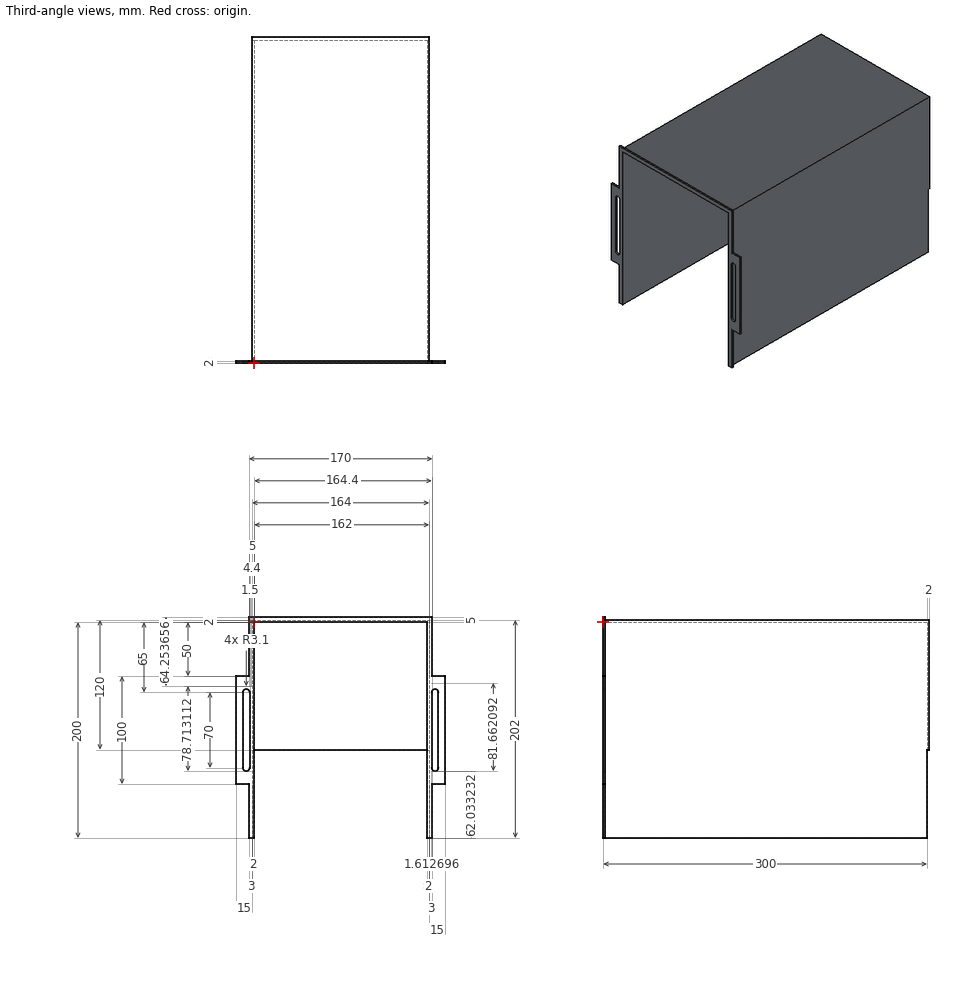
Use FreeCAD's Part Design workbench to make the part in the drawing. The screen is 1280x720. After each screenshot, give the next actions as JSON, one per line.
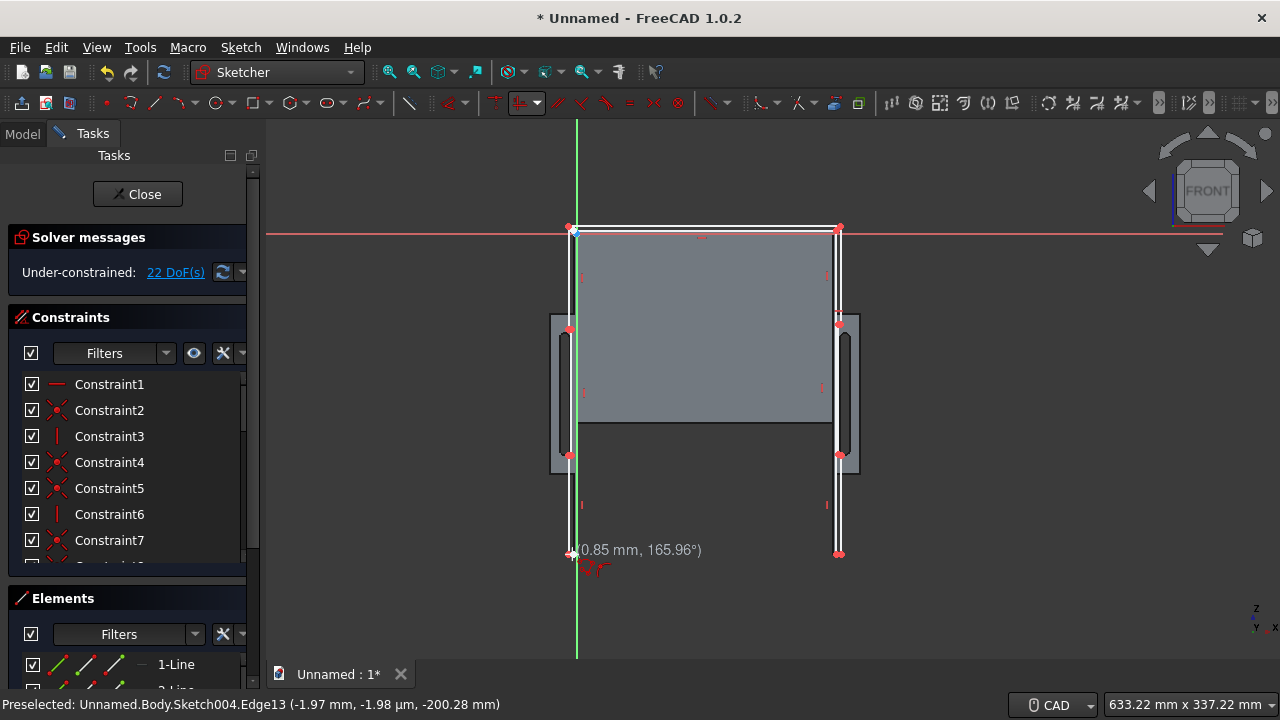
{"action": "scroll", "coordinate": [574, 231], "scroll_direction": "up", "scroll_amount": 9}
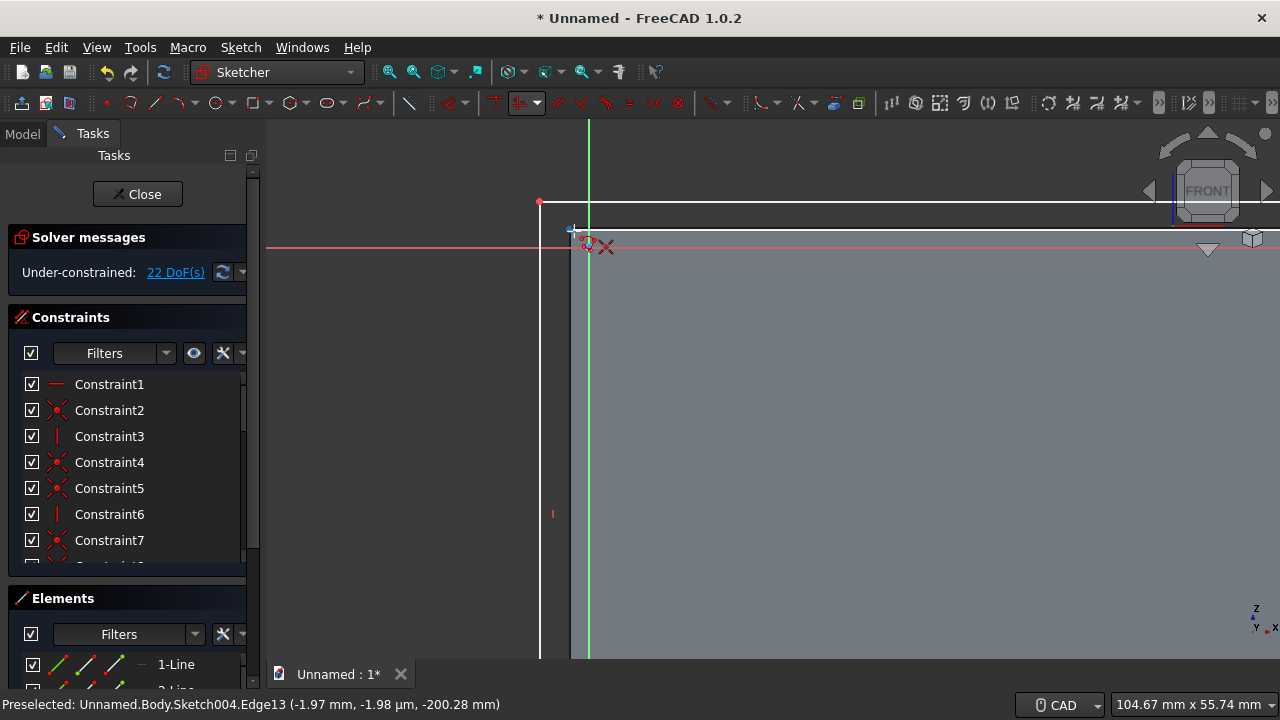
{"action": "left_click", "coordinate": [569, 230]}
{"action": "key", "text": "Escape"}
{"action": "key", "text": "Escape"}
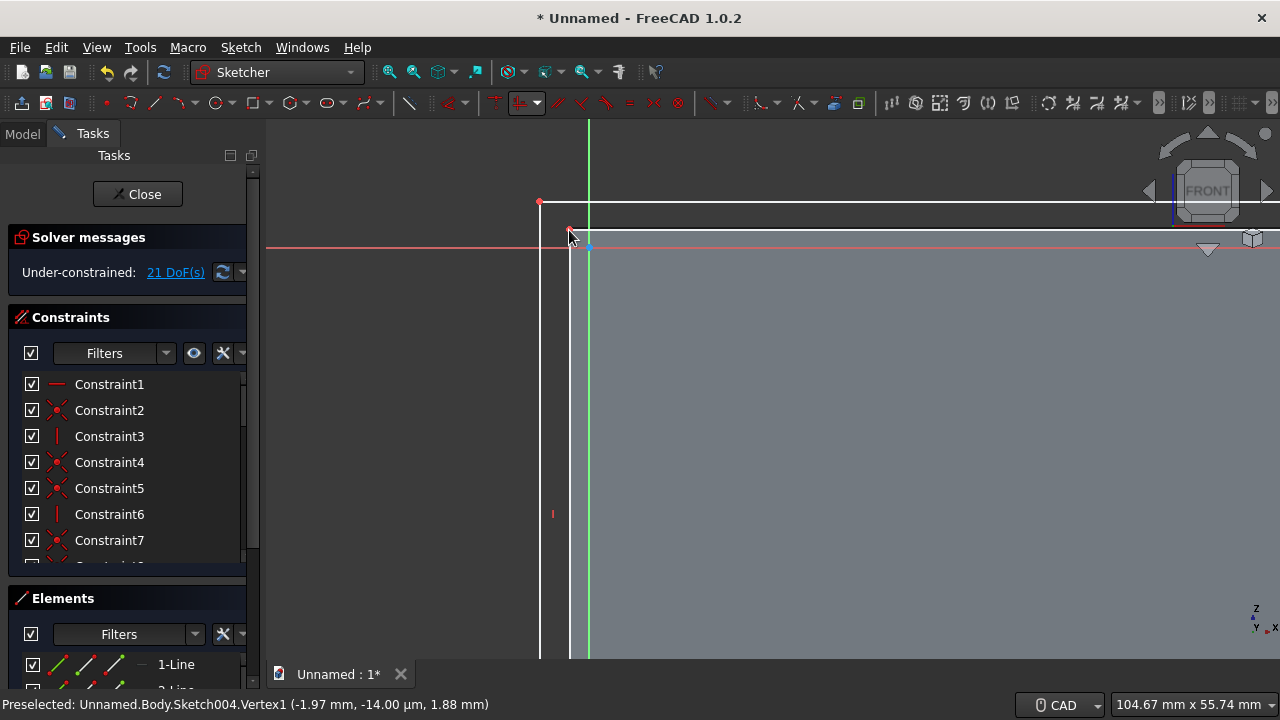
{"action": "scroll", "coordinate": [574, 230], "scroll_direction": "down", "scroll_amount": 9}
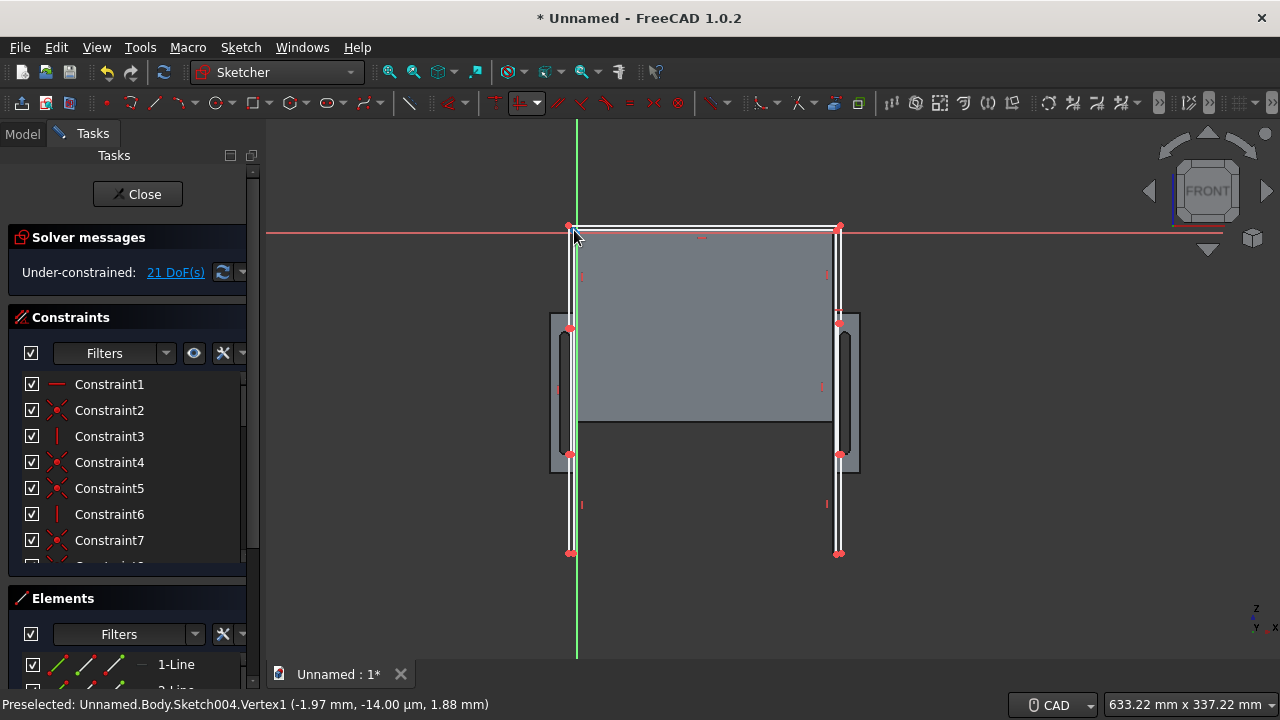
{"action": "scroll", "coordinate": [838, 554], "scroll_direction": "up", "scroll_amount": 10}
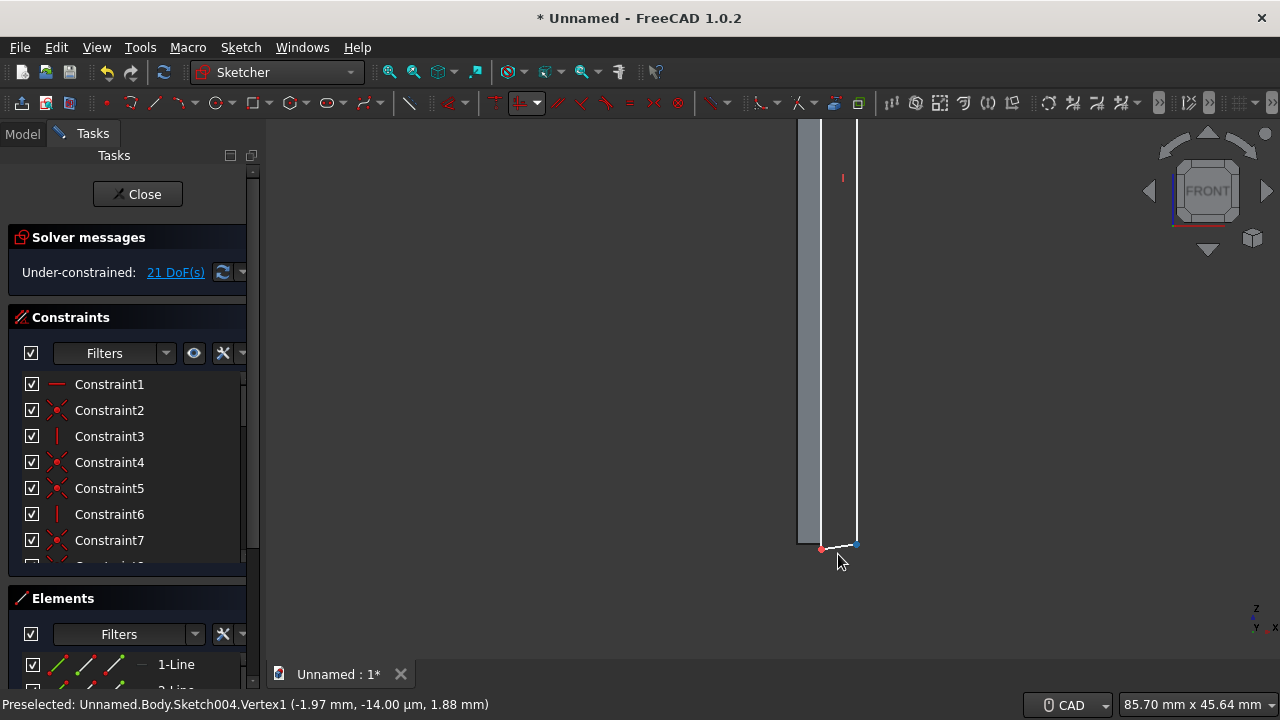
{"action": "left_click", "coordinate": [836, 547]}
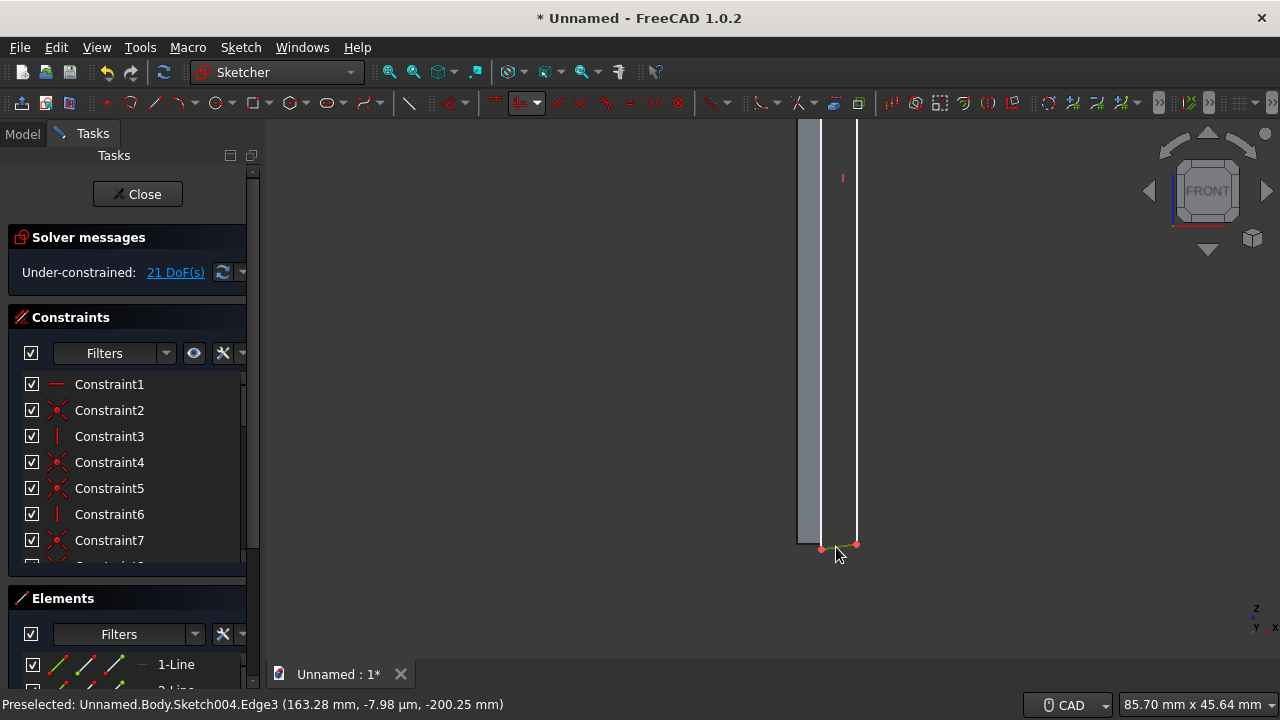
{"action": "key", "text": "h"}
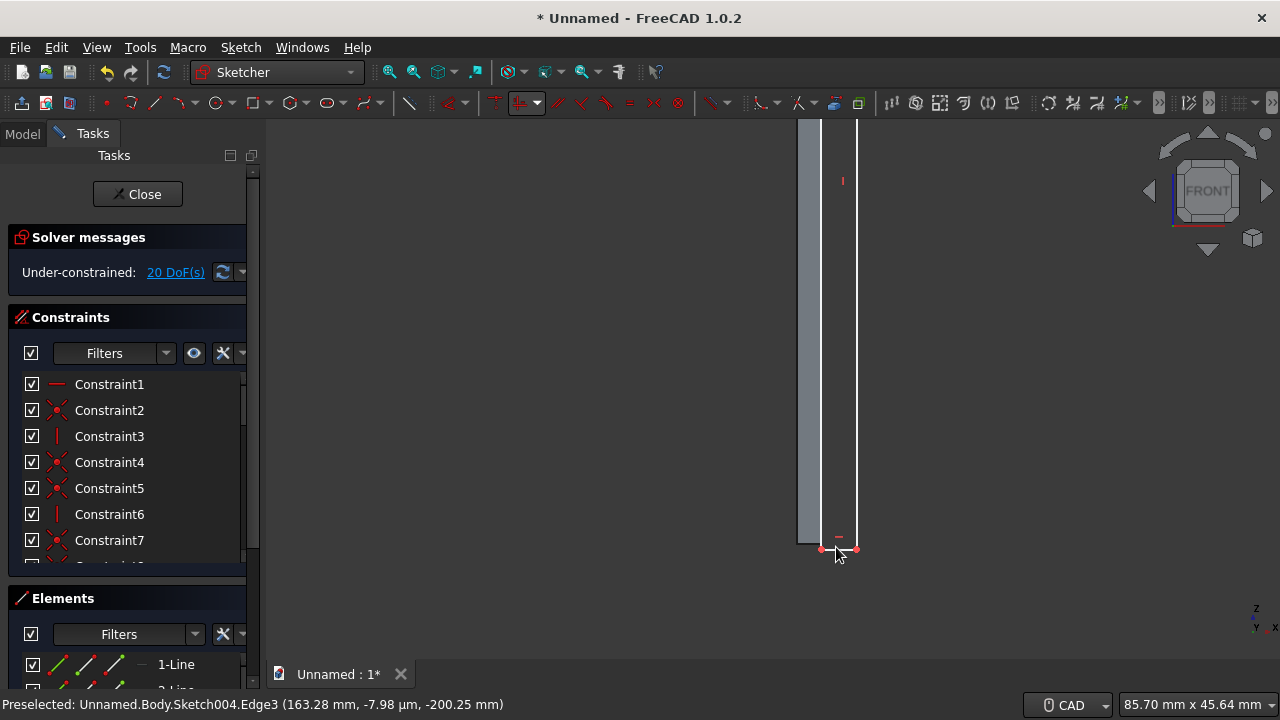
{"action": "scroll", "coordinate": [838, 555], "scroll_direction": "down", "scroll_amount": 10}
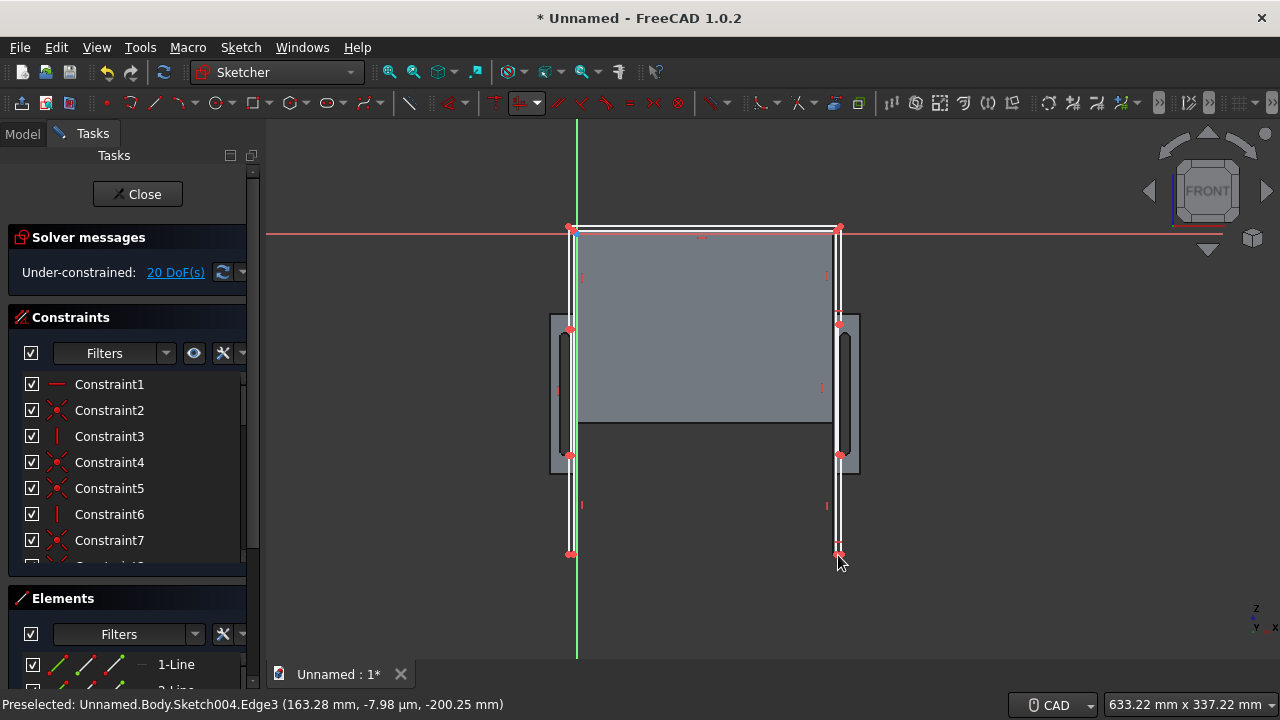
{"action": "scroll", "coordinate": [840, 455], "scroll_direction": "up", "scroll_amount": 12}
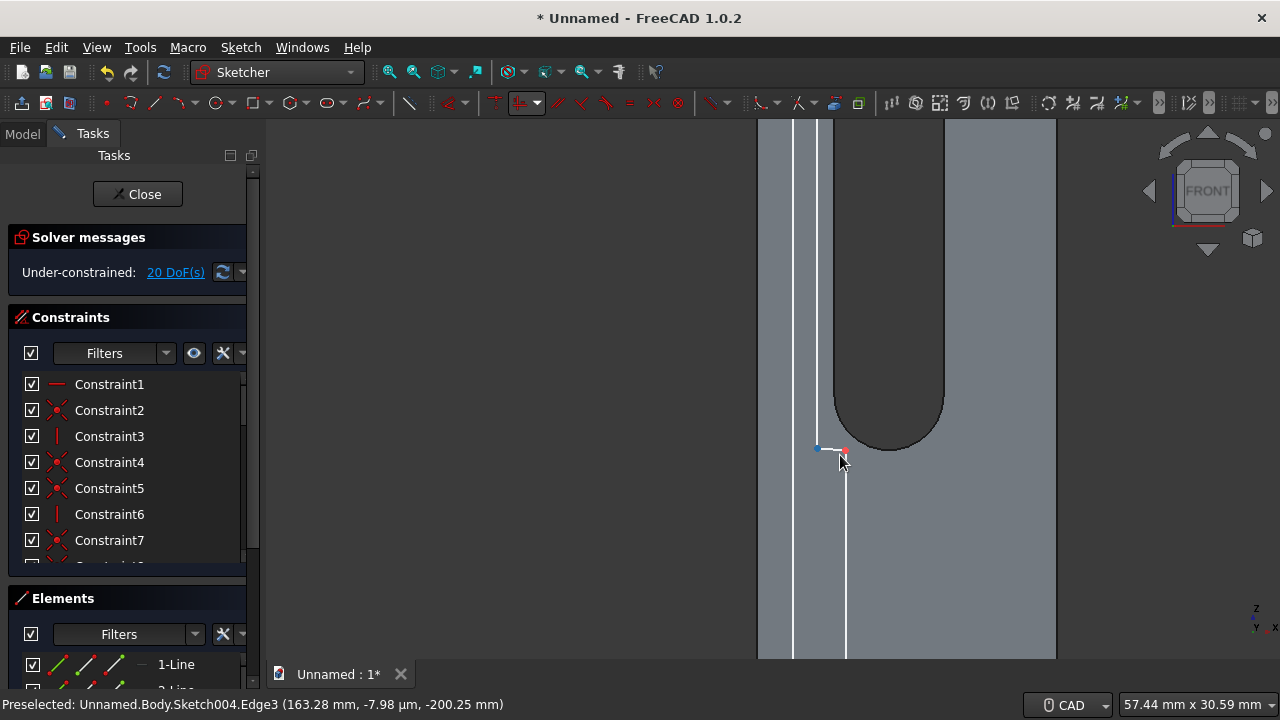
{"action": "left_click", "coordinate": [831, 449]}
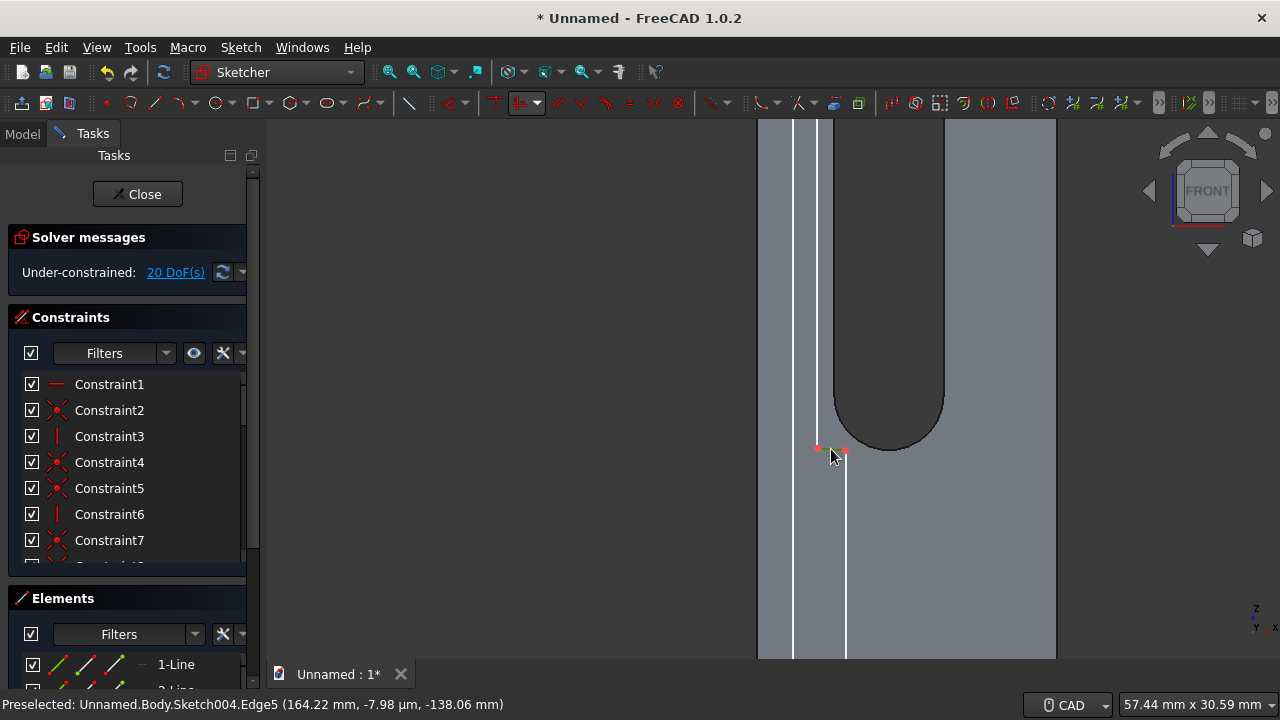
{"action": "left_click", "coordinate": [540, 104]}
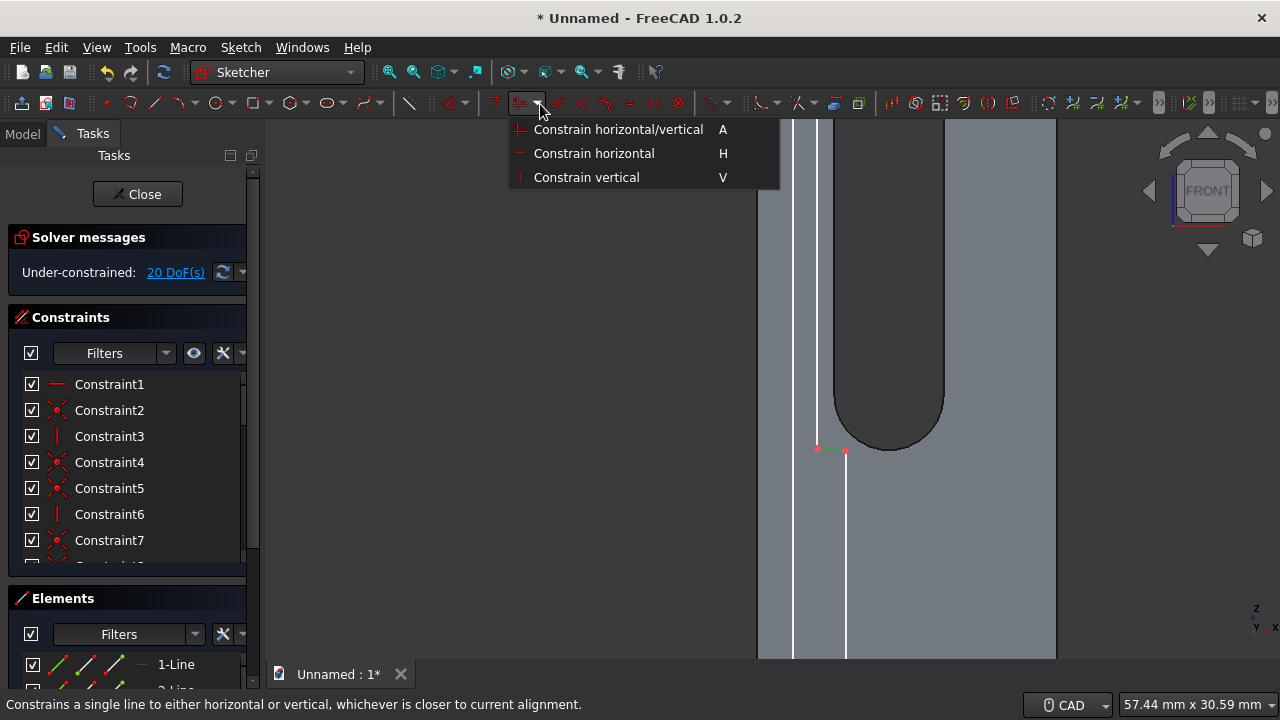
{"action": "left_click", "coordinate": [644, 153]}